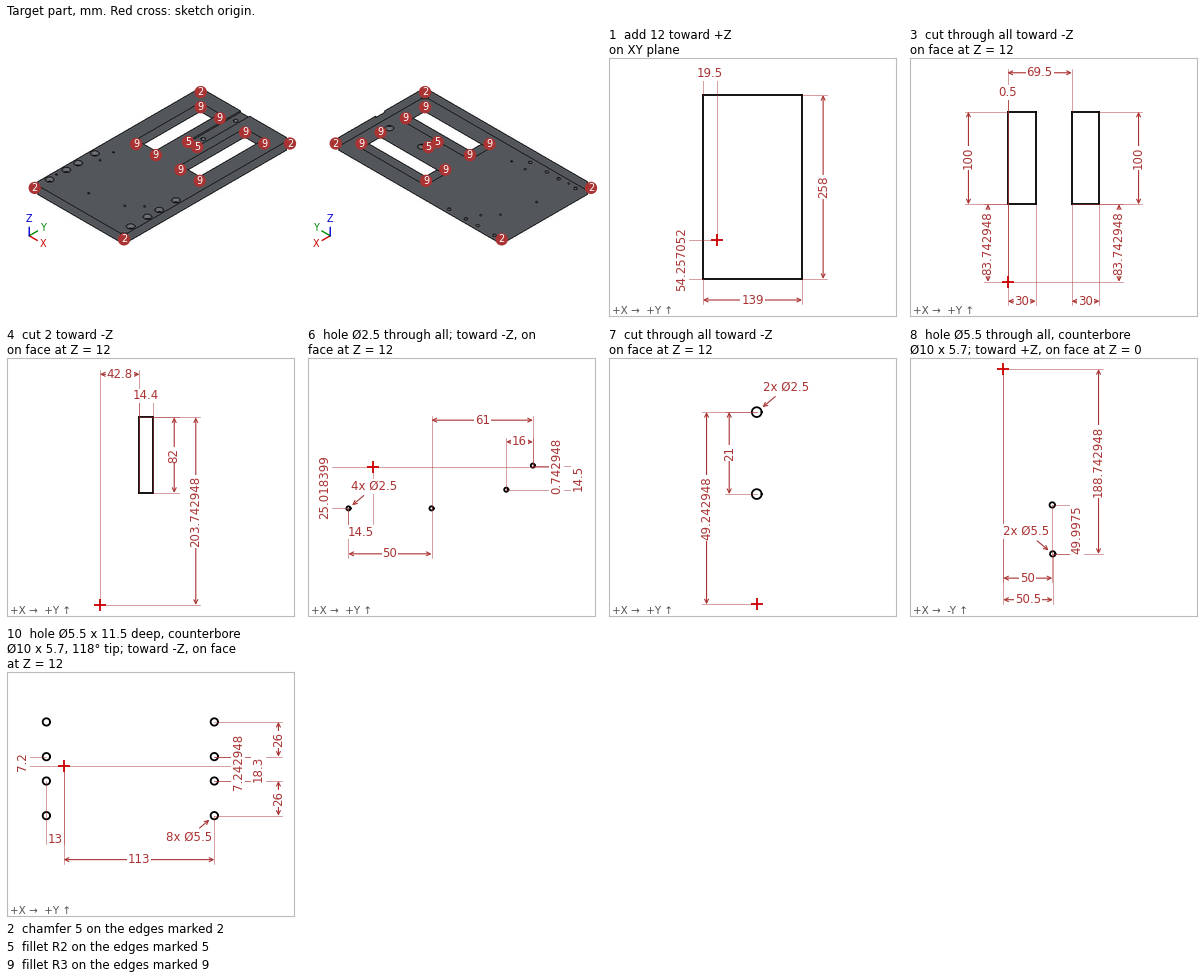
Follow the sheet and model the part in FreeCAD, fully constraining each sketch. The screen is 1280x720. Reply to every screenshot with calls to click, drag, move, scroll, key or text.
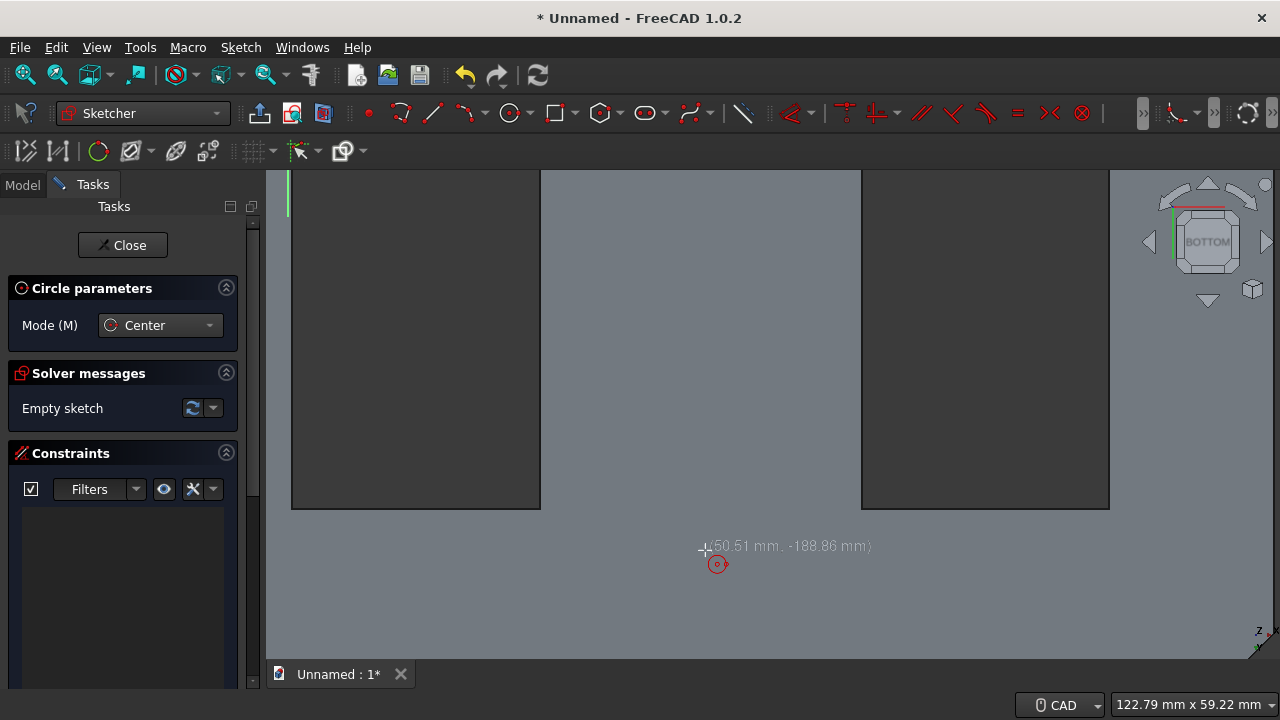
click(705, 550)
move(721, 534)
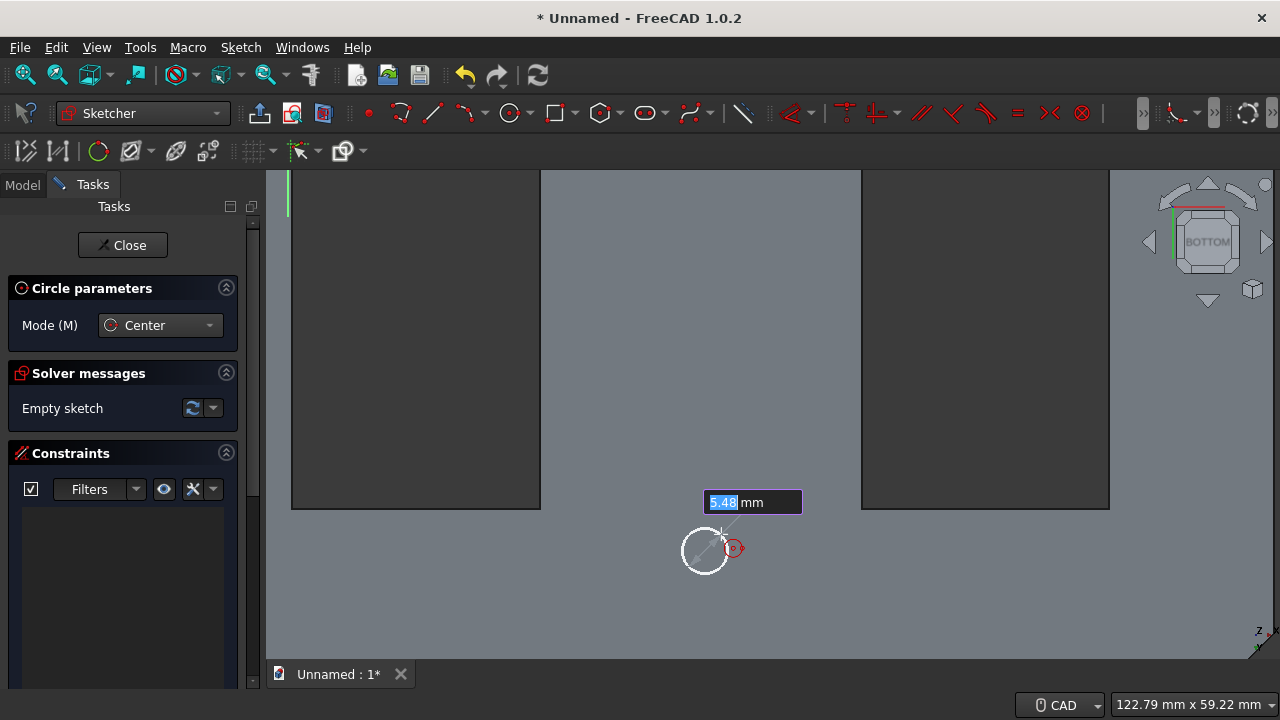
text(5.5)
key(Return)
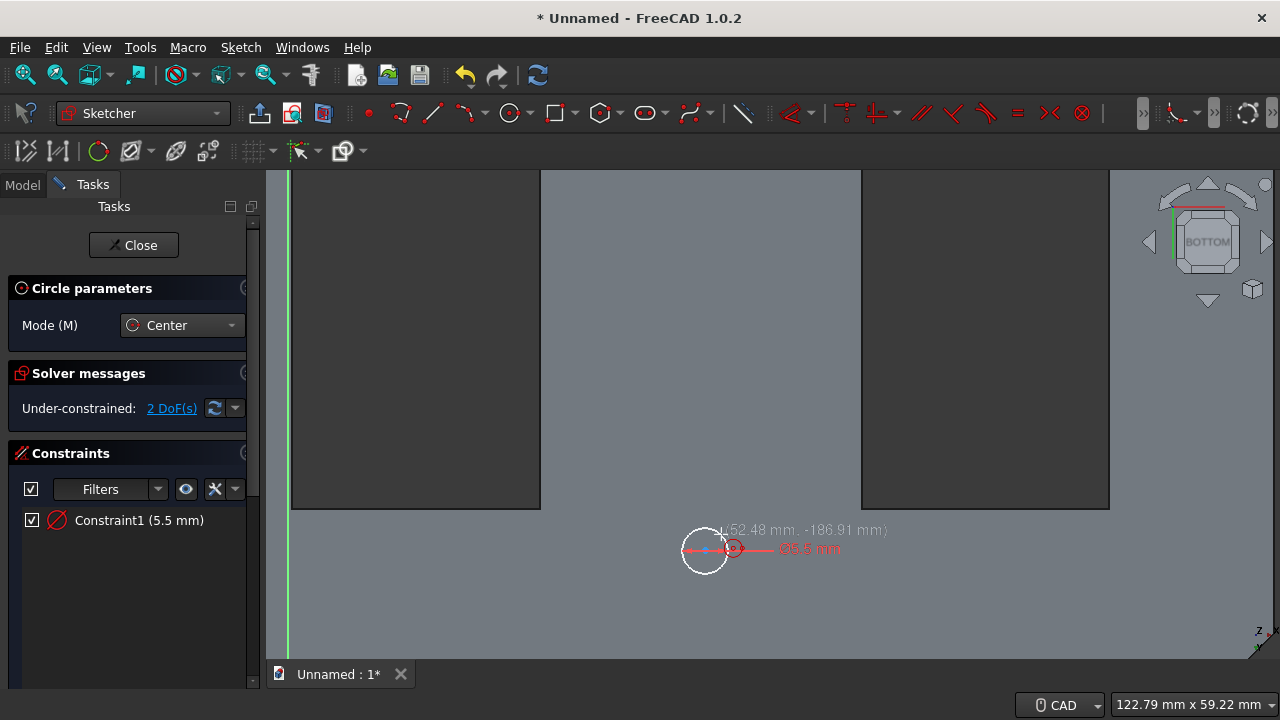
scroll(708, 559, down, 2)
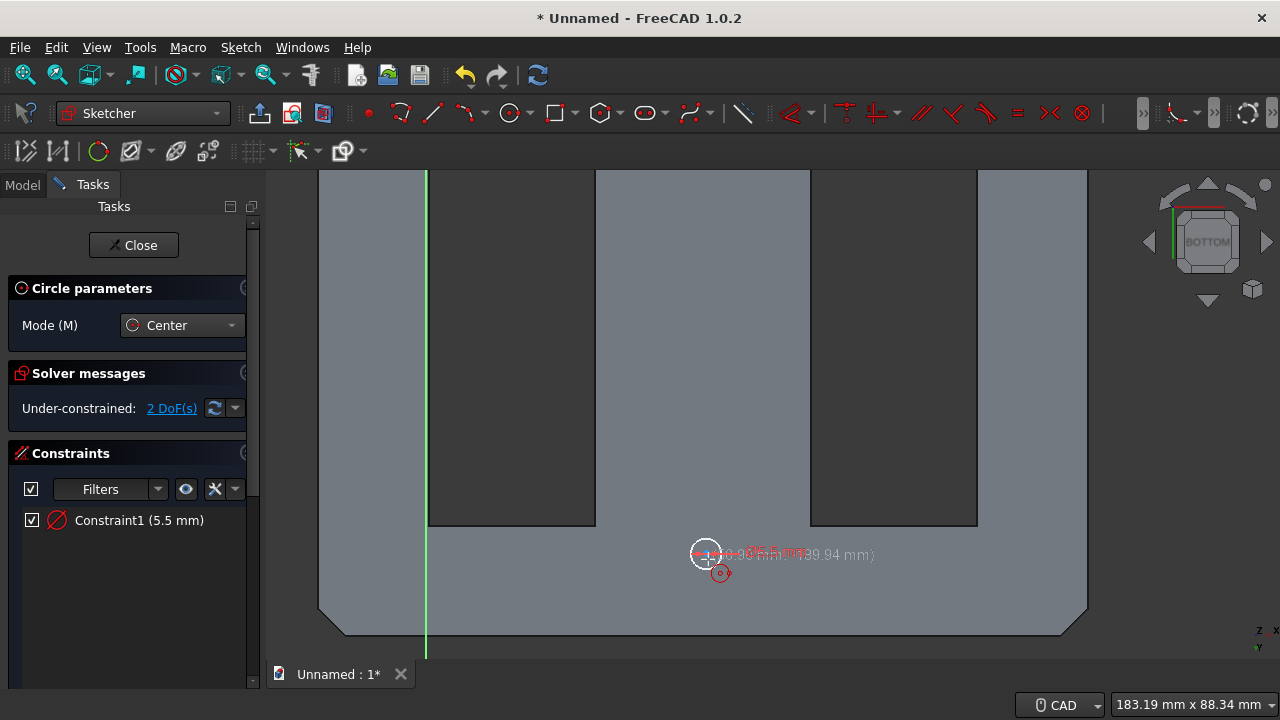
scroll(703, 277, up, 2)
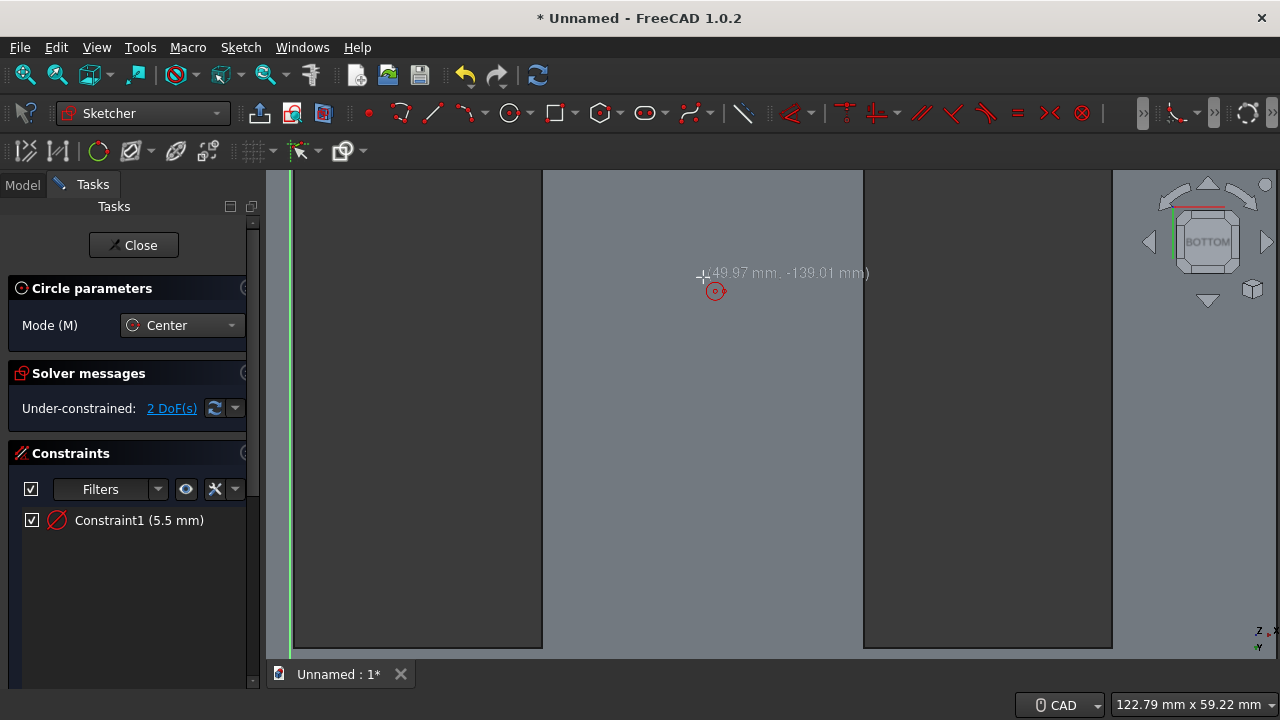
click(703, 276)
move(719, 260)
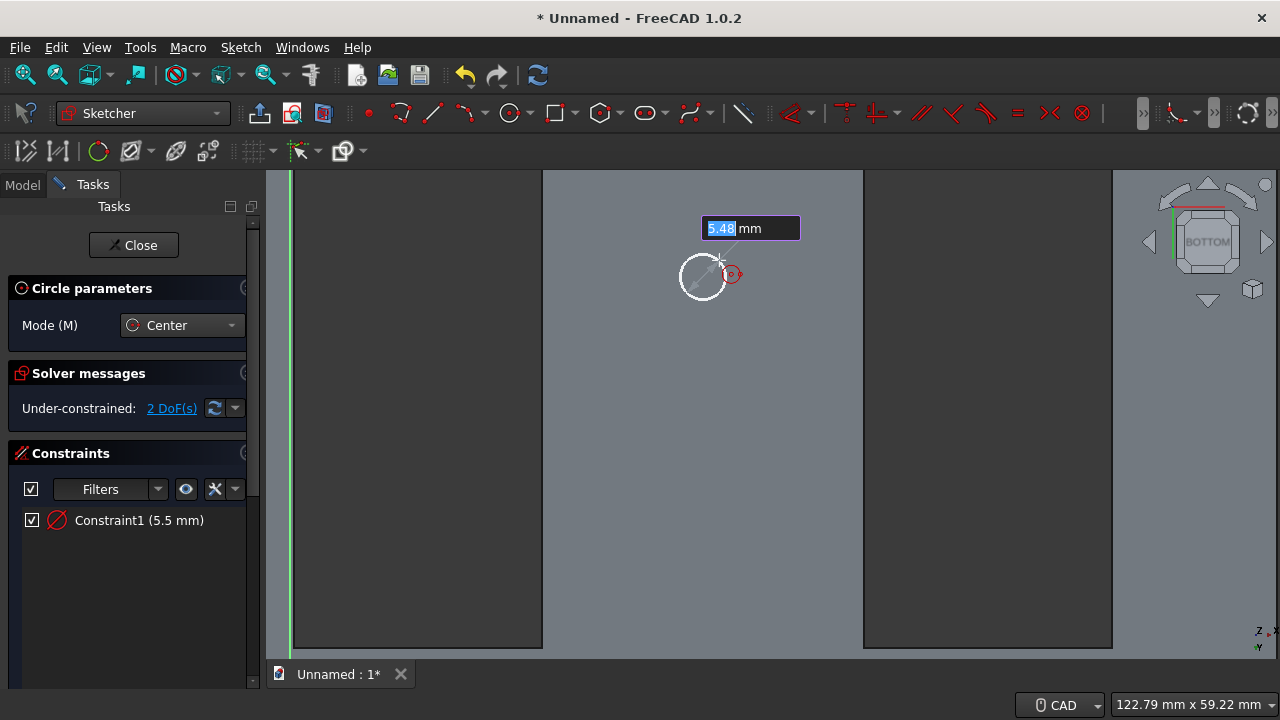
text(5.5)
key(Return)
key(Escape)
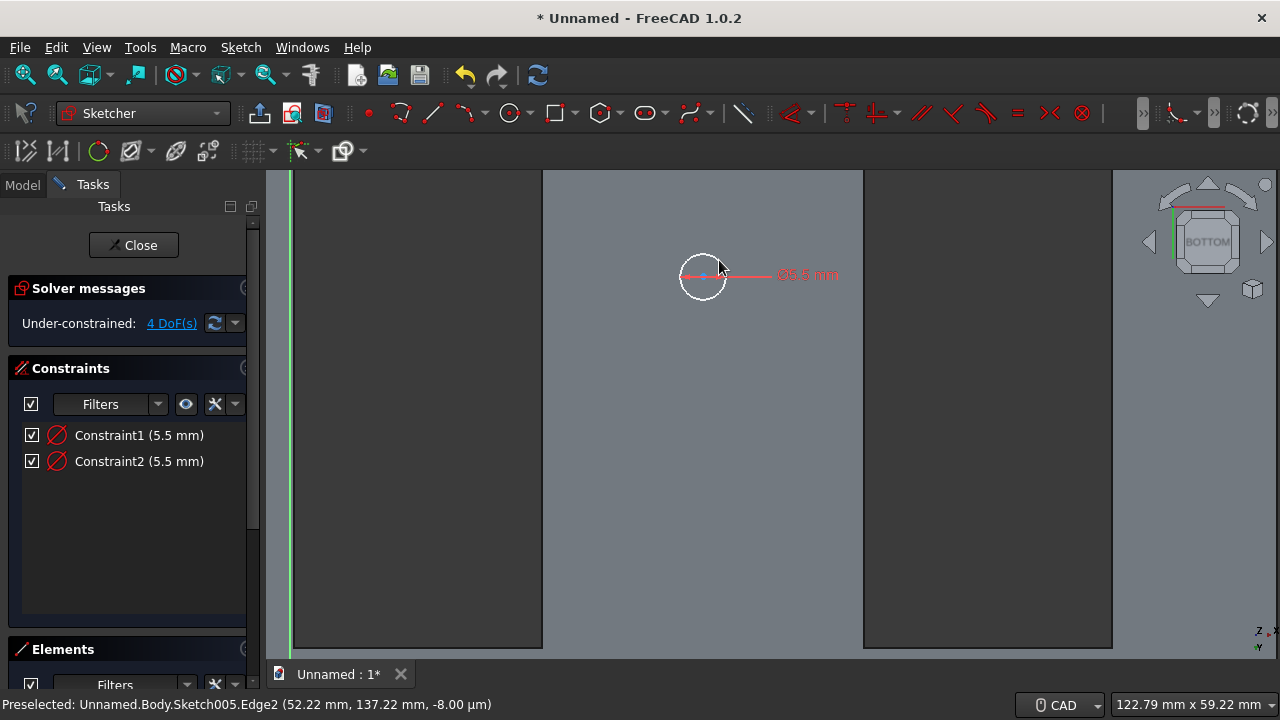
click(790, 114)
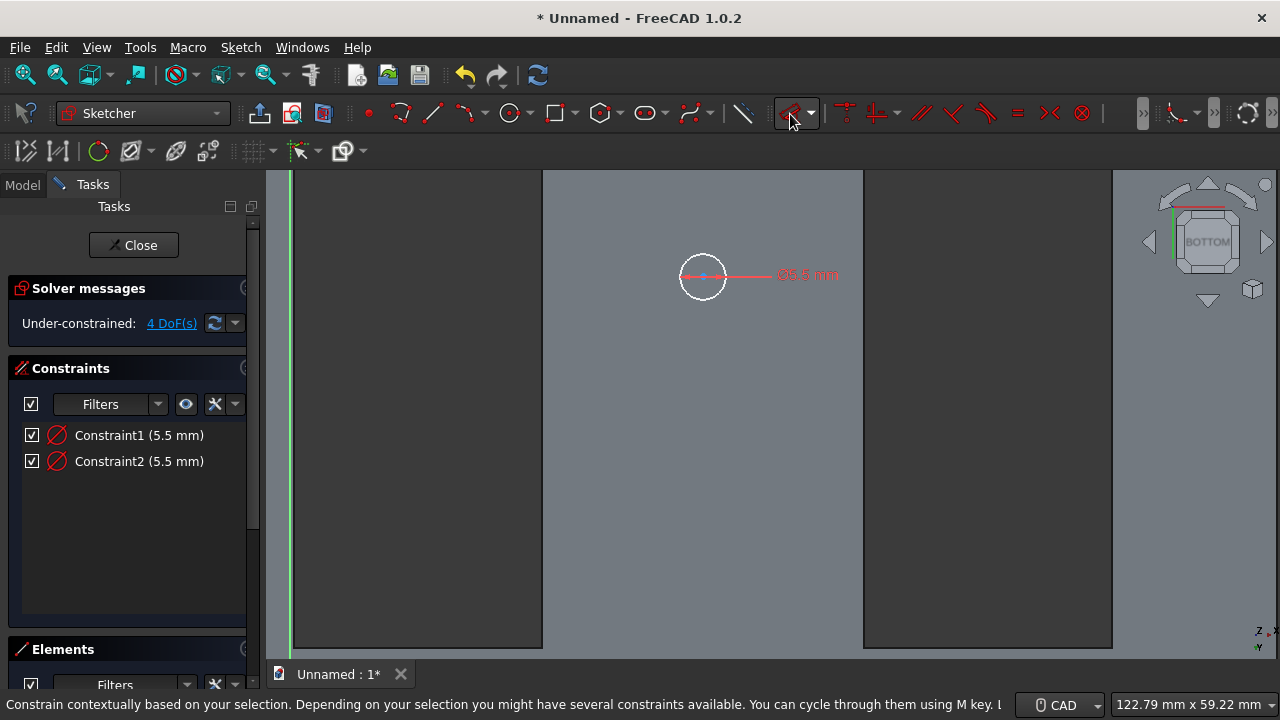
click(703, 277)
click(498, 311)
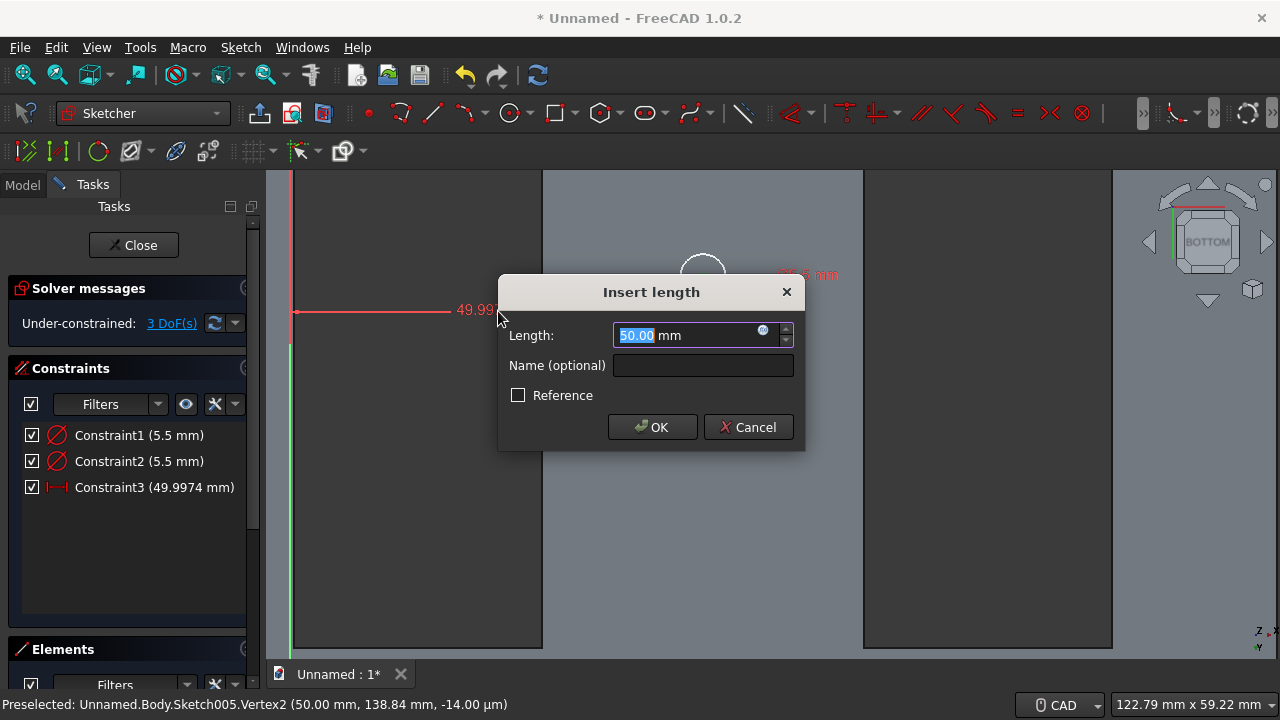
text(50)
key(Return)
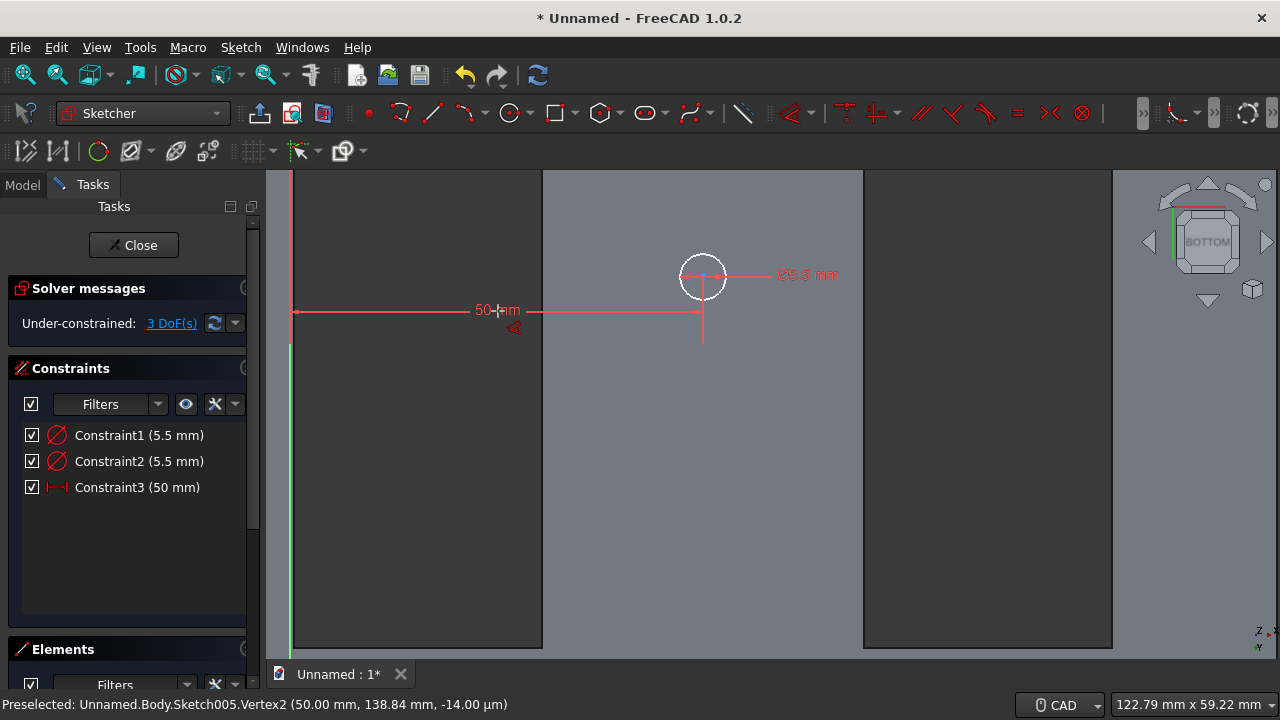
scroll(703, 276, down, 2)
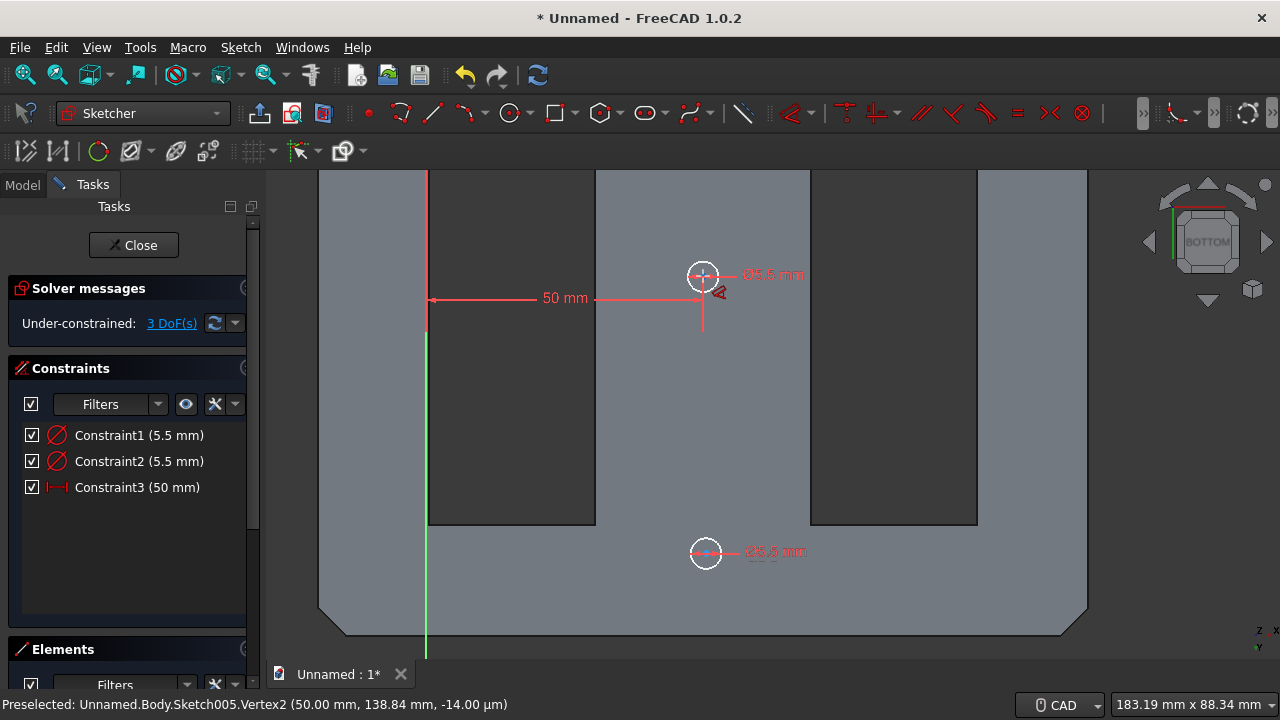
click(706, 554)
click(566, 588)